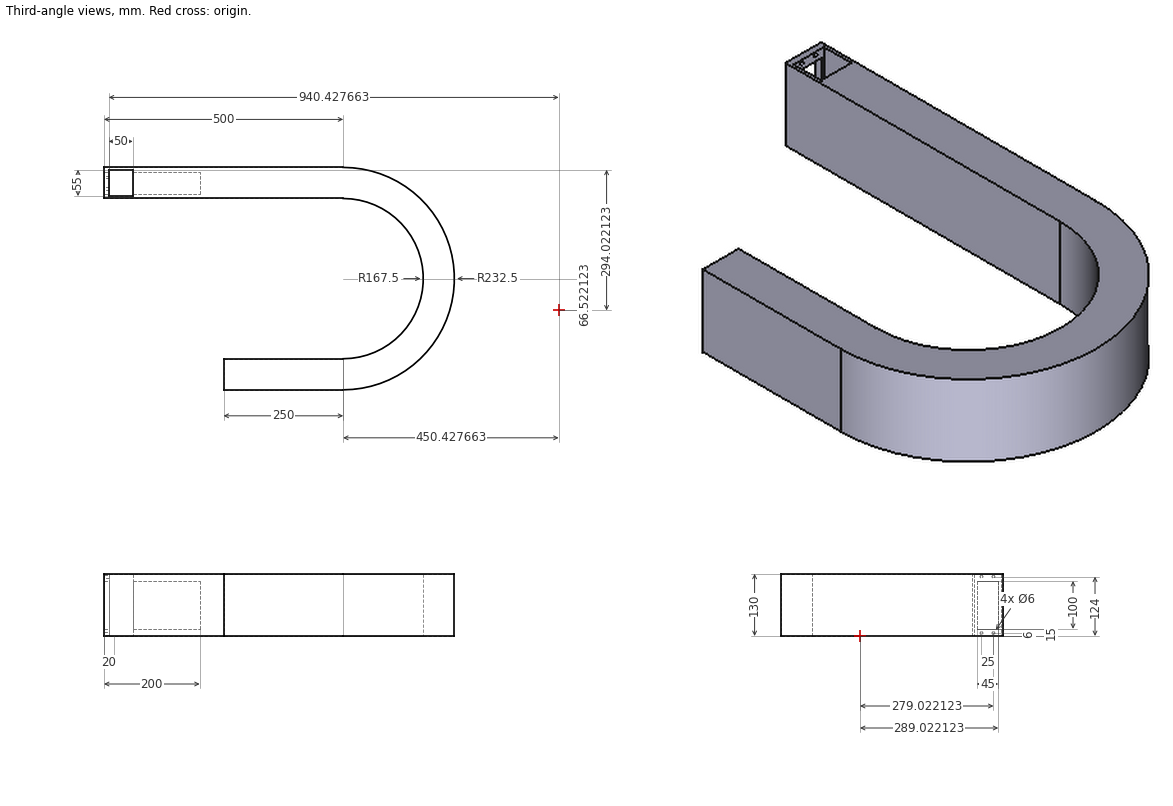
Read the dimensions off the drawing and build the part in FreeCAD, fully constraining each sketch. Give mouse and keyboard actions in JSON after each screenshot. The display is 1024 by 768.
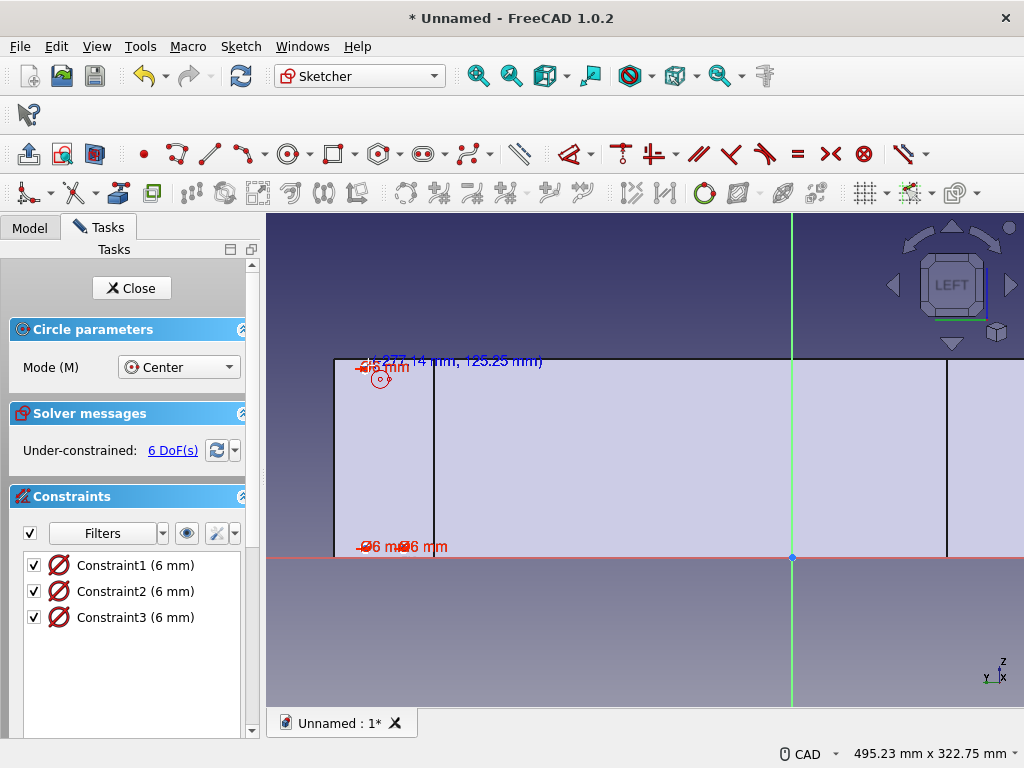
{"action": "scroll", "coordinate": [403, 368], "scroll_direction": "up", "scroll_amount": 8}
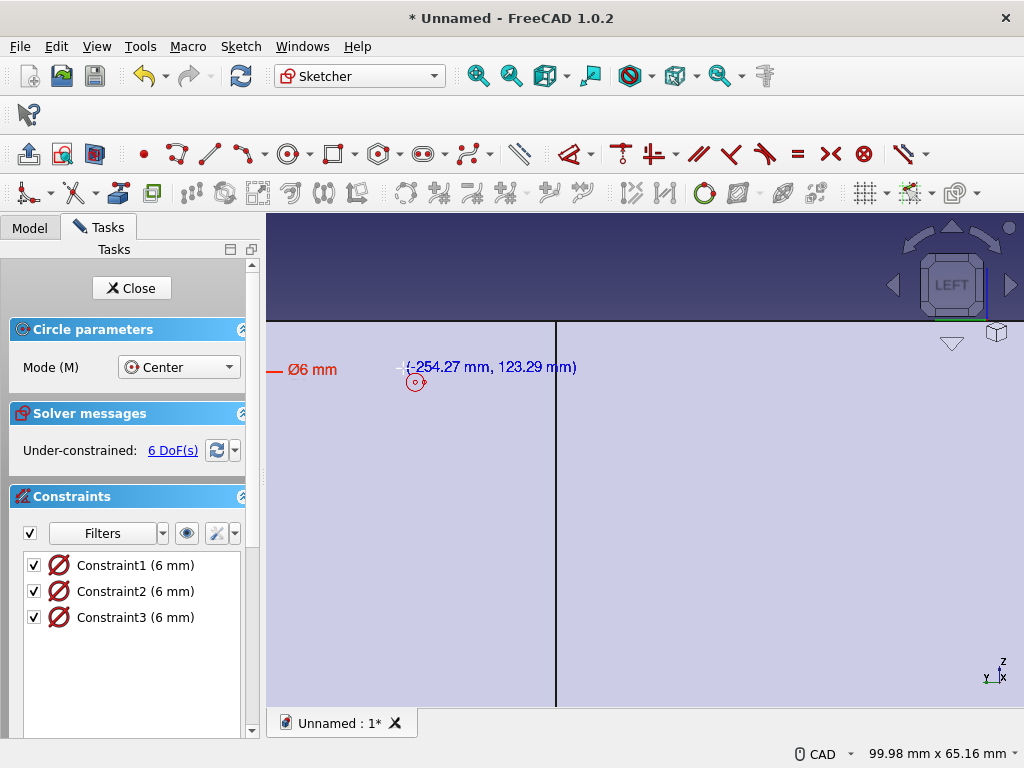
{"action": "scroll", "coordinate": [403, 368], "scroll_direction": "down", "scroll_amount": 8}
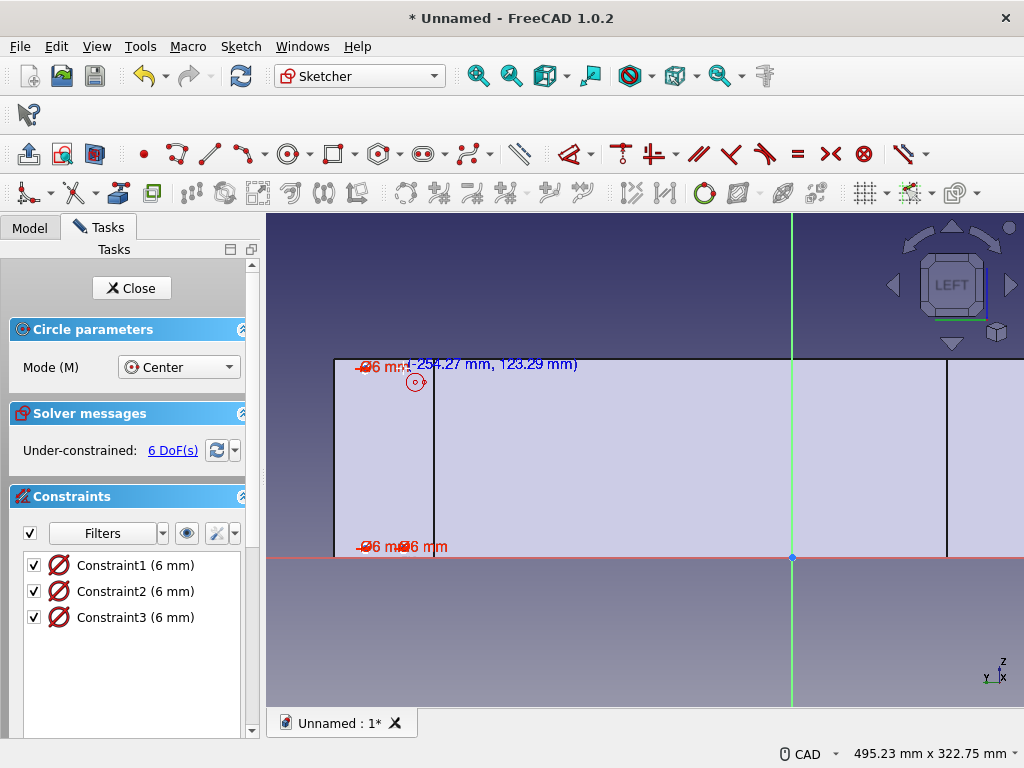
{"action": "left_click", "coordinate": [403, 368]}
{"action": "mouse_move", "coordinate": [407, 365]}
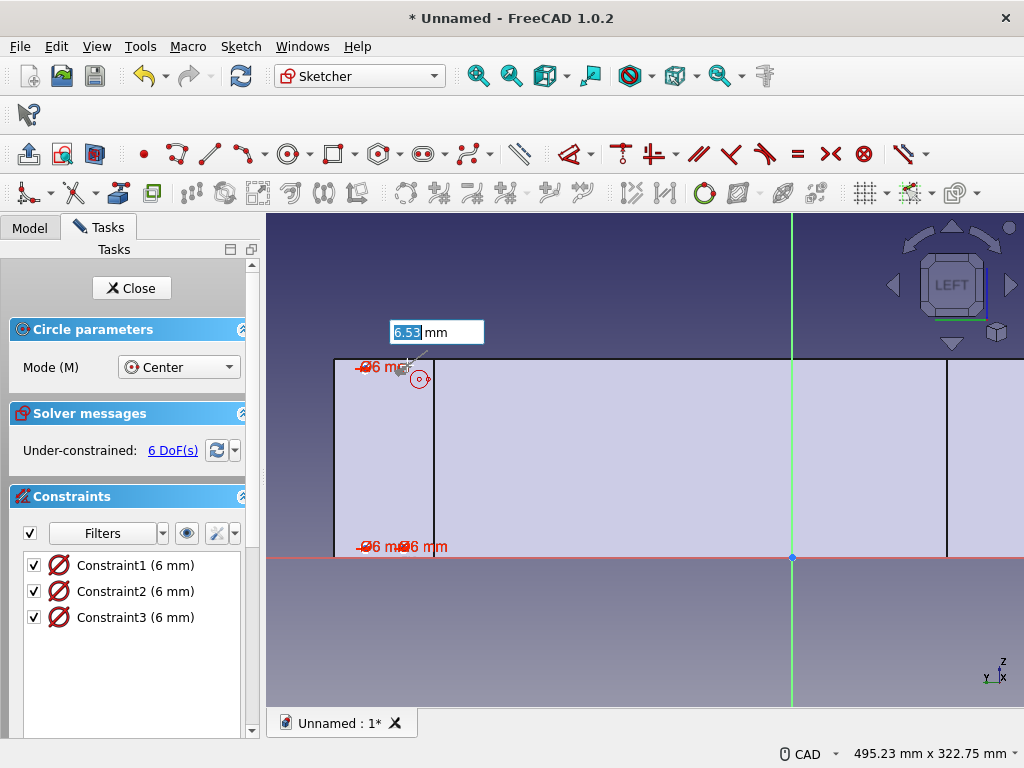
{"action": "type", "text": "6"}
{"action": "key", "text": "Return"}
{"action": "key", "text": "Escape"}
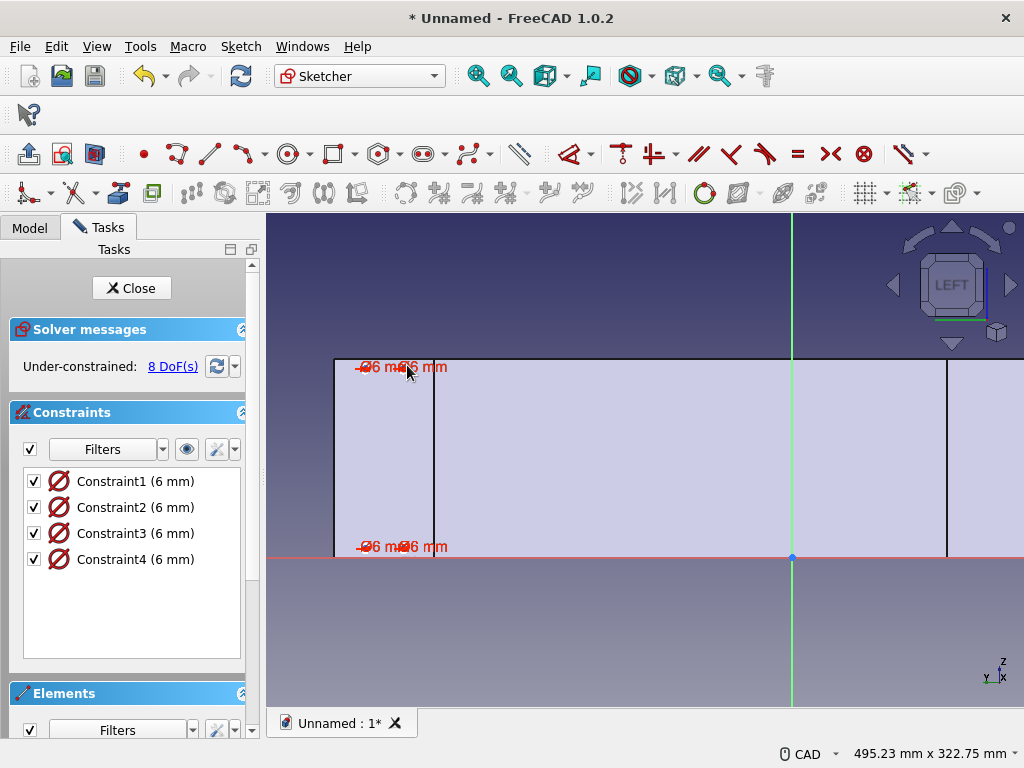
{"action": "key", "text": "d"}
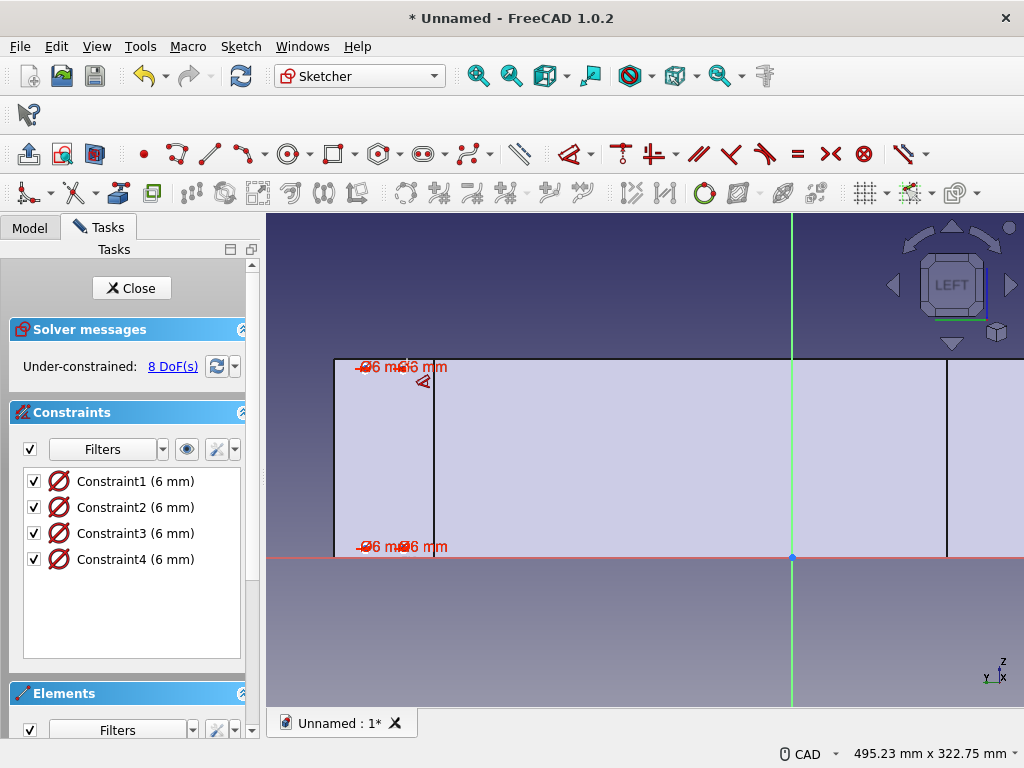
{"action": "scroll", "coordinate": [365, 549], "scroll_direction": "up", "scroll_amount": 8}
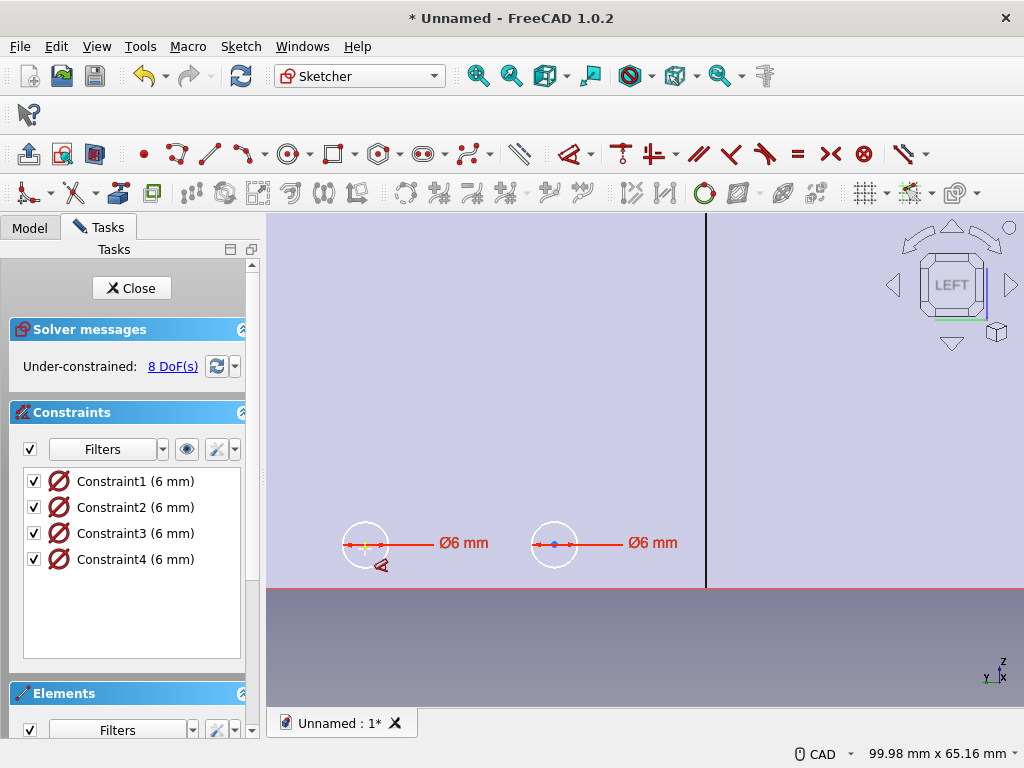
{"action": "left_click", "coordinate": [365, 545]}
{"action": "left_click", "coordinate": [331, 567]}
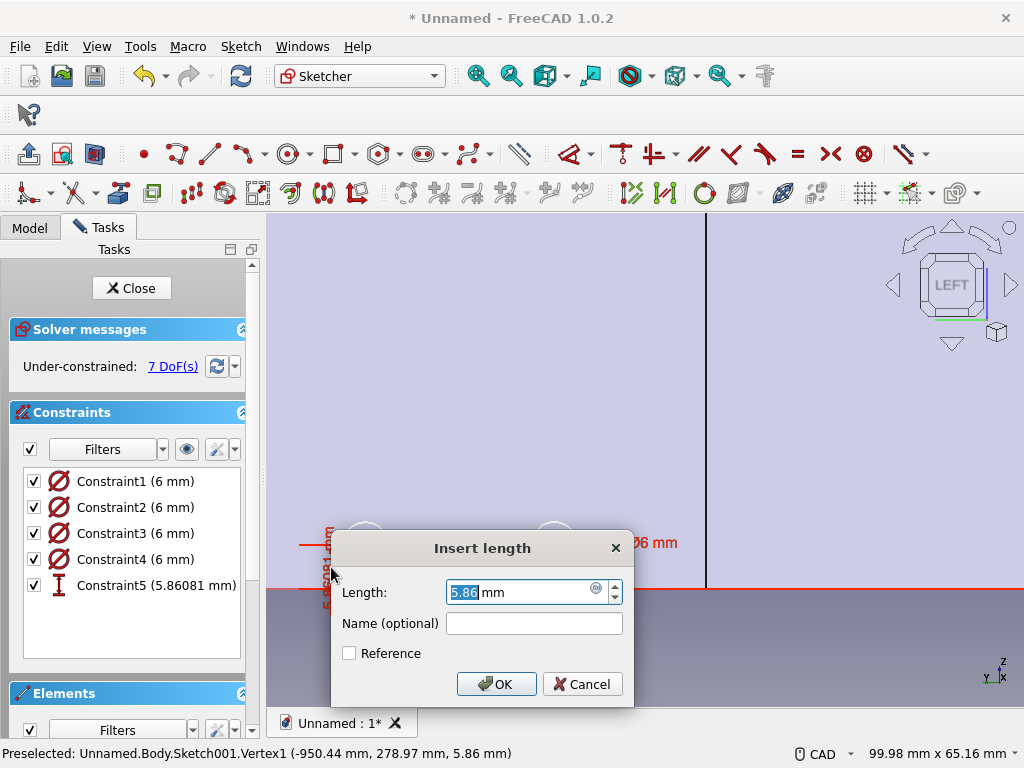
{"action": "type", "text": "6"}
{"action": "key", "text": "Return"}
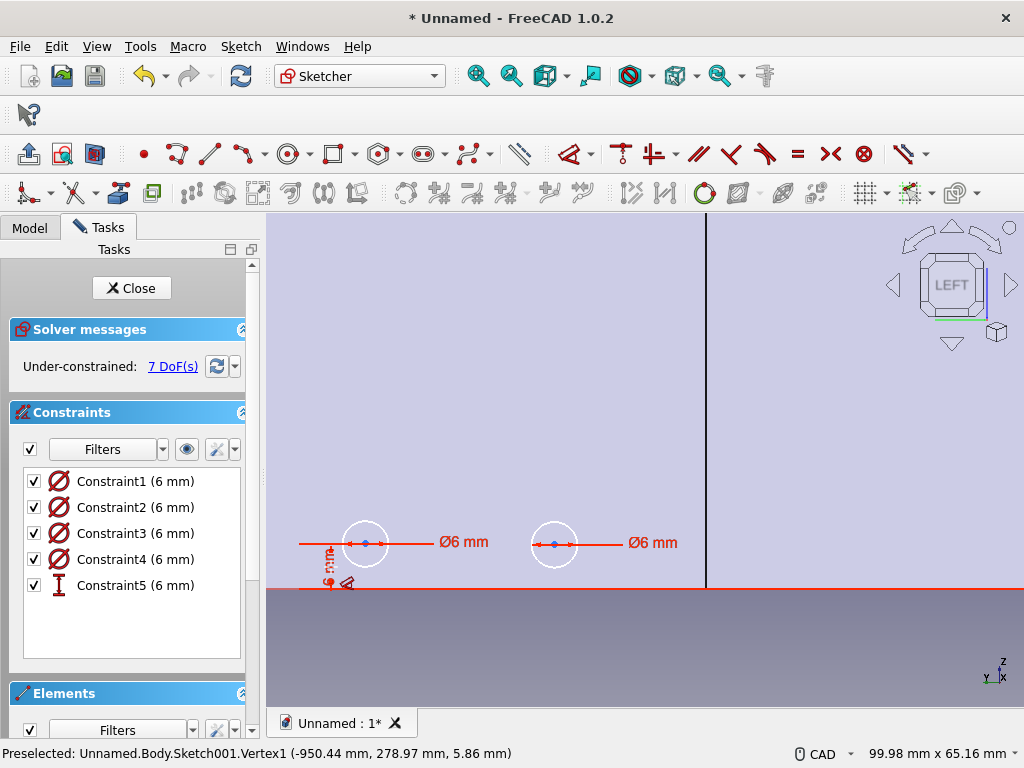
{"action": "left_click", "coordinate": [554, 545]}
{"action": "left_click", "coordinate": [520, 567]}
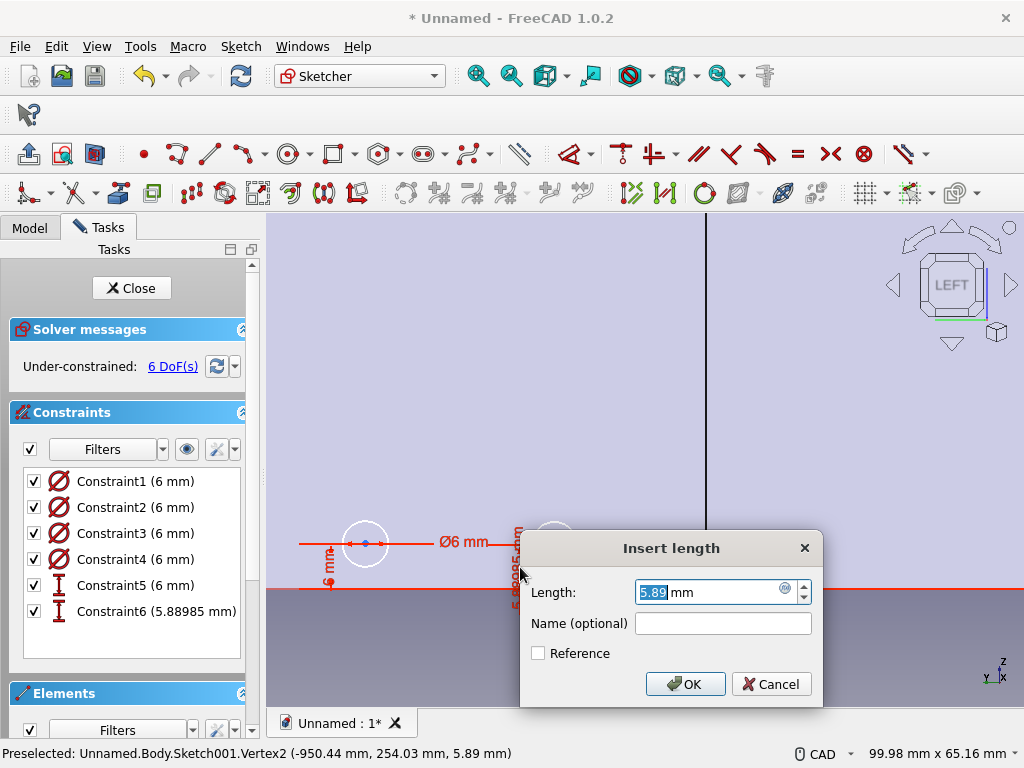
{"action": "type", "text": "6"}
{"action": "key", "text": "Return"}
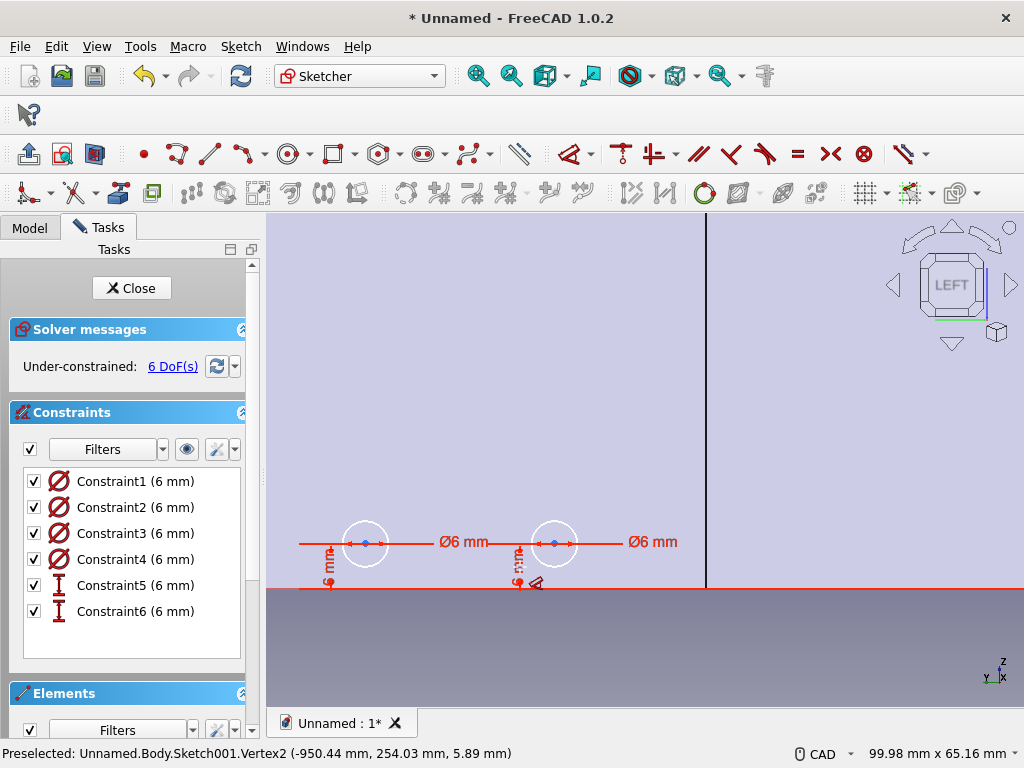
{"action": "scroll", "coordinate": [365, 549], "scroll_direction": "down", "scroll_amount": 8}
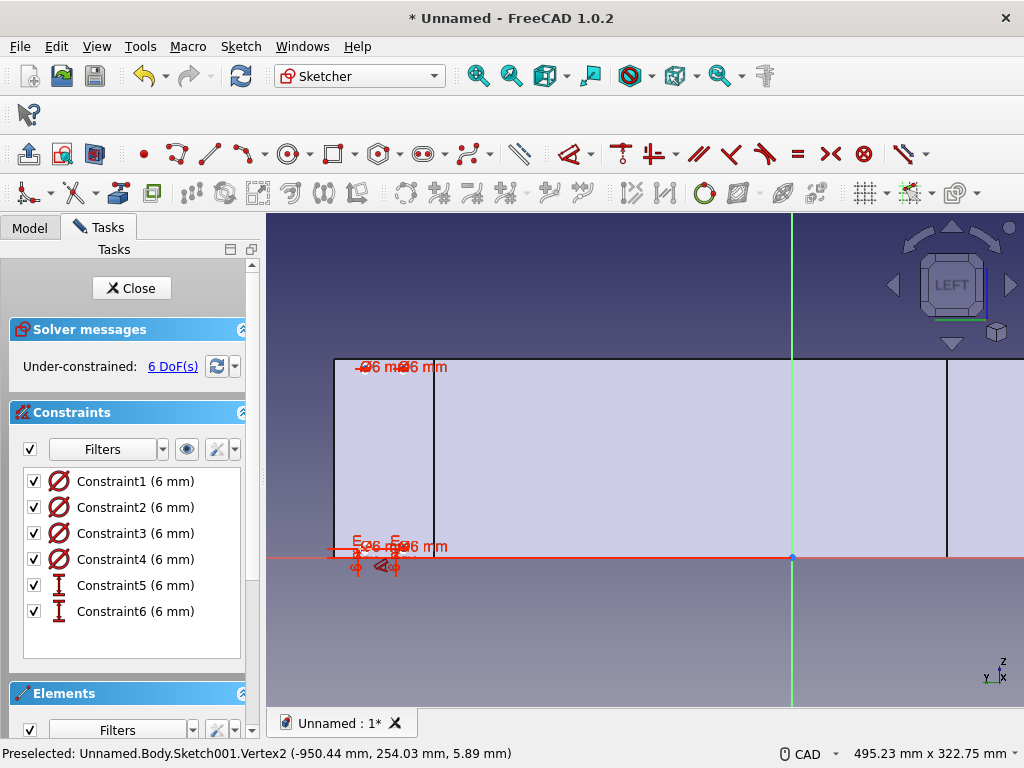
{"action": "left_click", "coordinate": [365, 369]}
{"action": "left_click", "coordinate": [826, 463]}